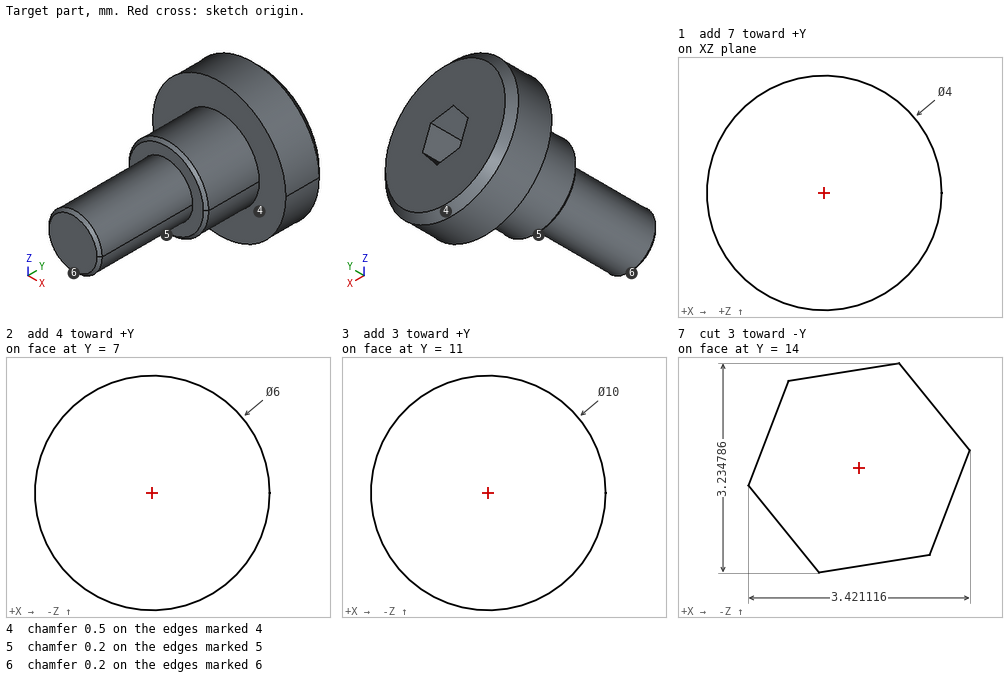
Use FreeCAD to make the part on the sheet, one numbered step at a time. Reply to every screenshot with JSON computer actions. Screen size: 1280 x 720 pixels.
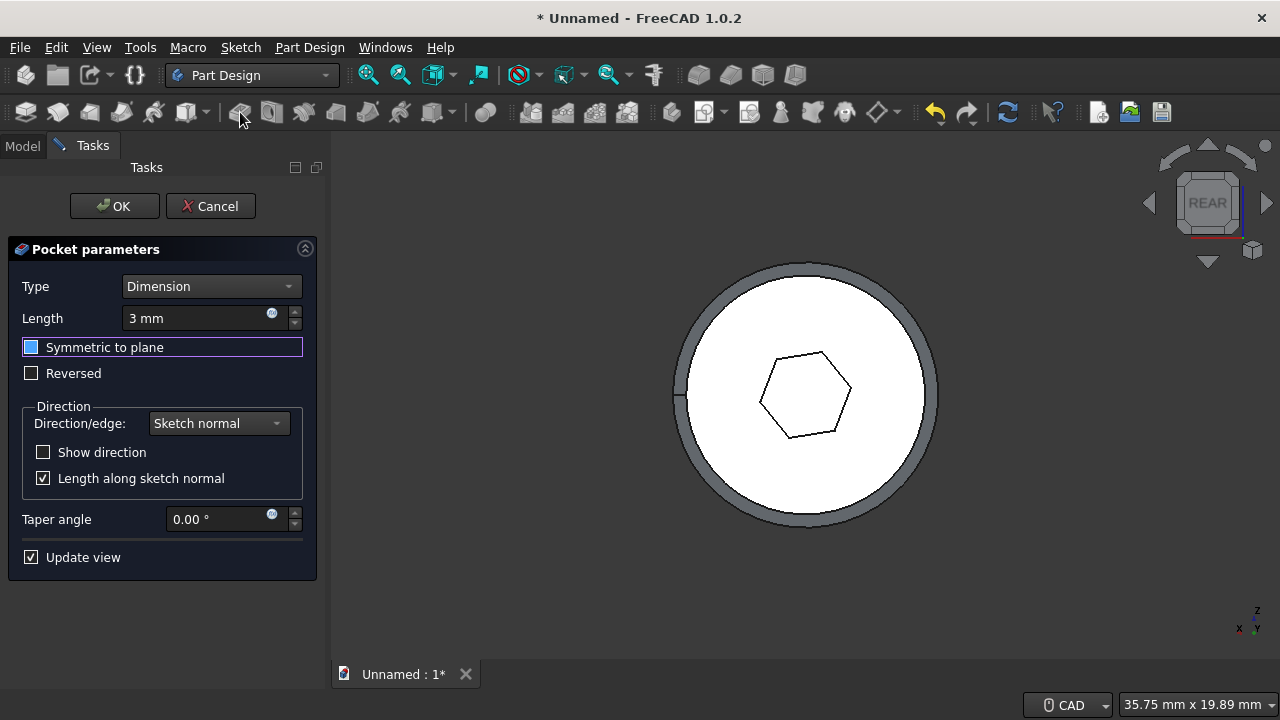
{"action": "left_click", "coordinate": [115, 206]}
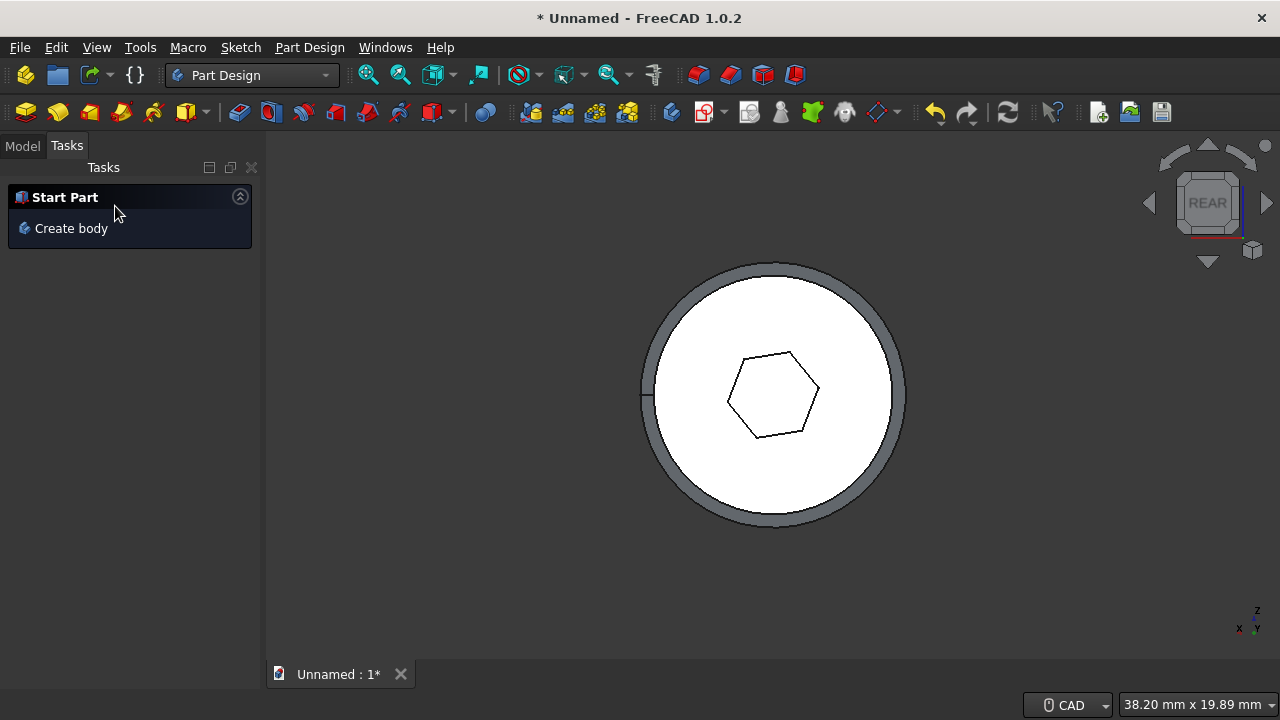
{"action": "key", "text": "0"}